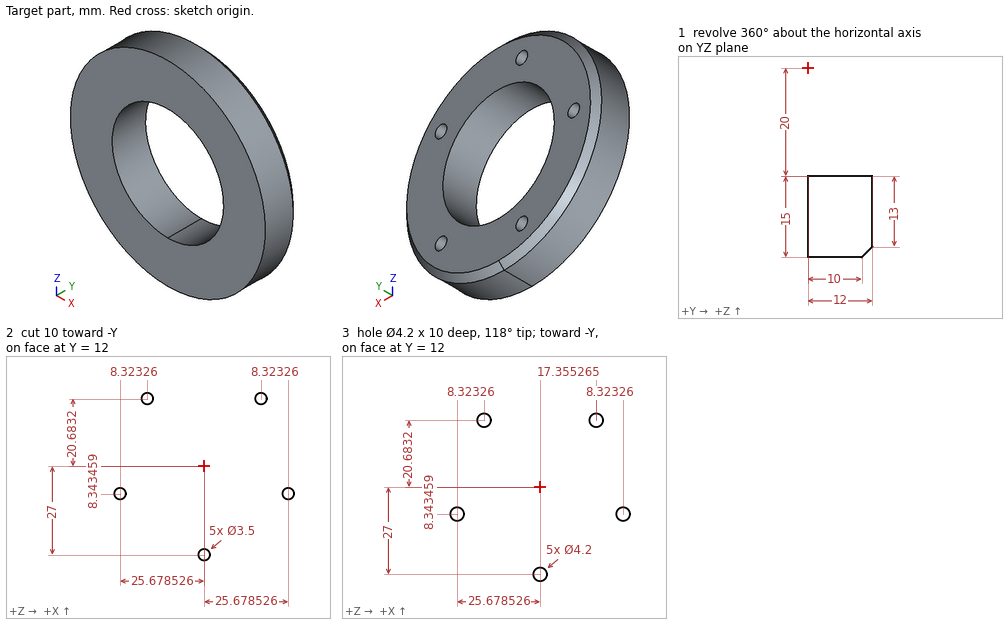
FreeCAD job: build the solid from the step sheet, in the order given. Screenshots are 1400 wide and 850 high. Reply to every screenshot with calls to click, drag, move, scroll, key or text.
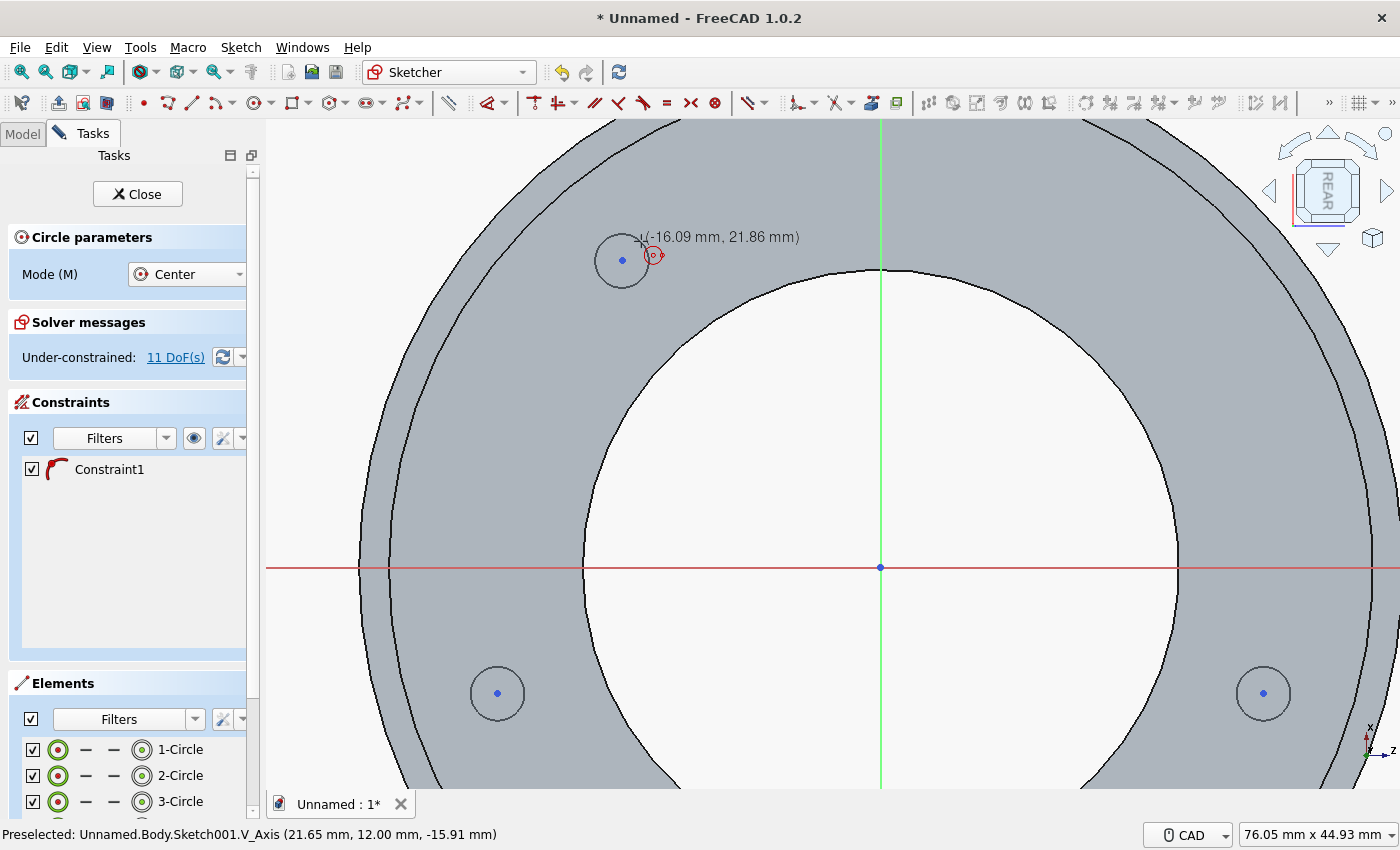
click(1140, 260)
click(1158, 241)
key(Escape)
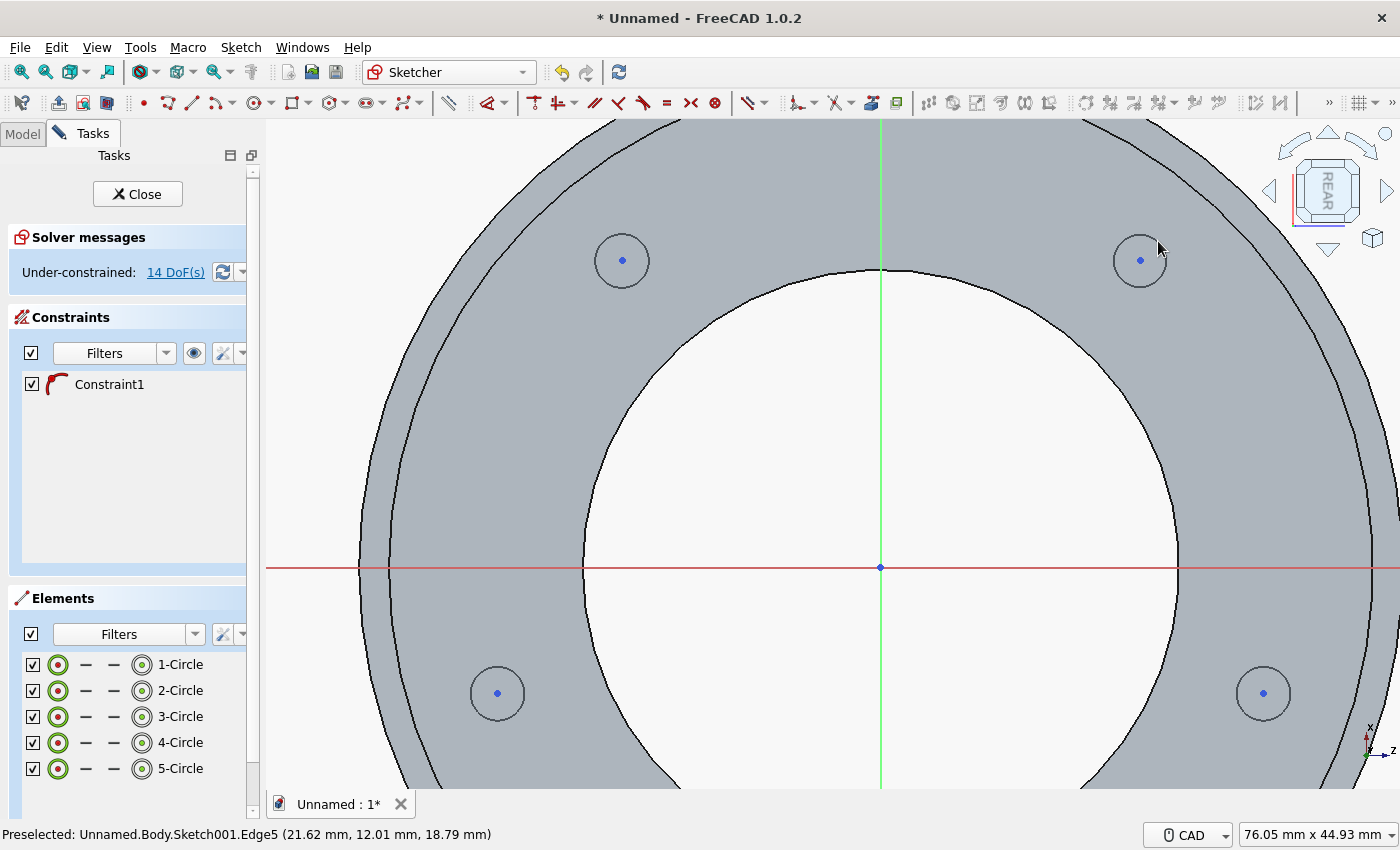
scroll(623, 258, down, 3)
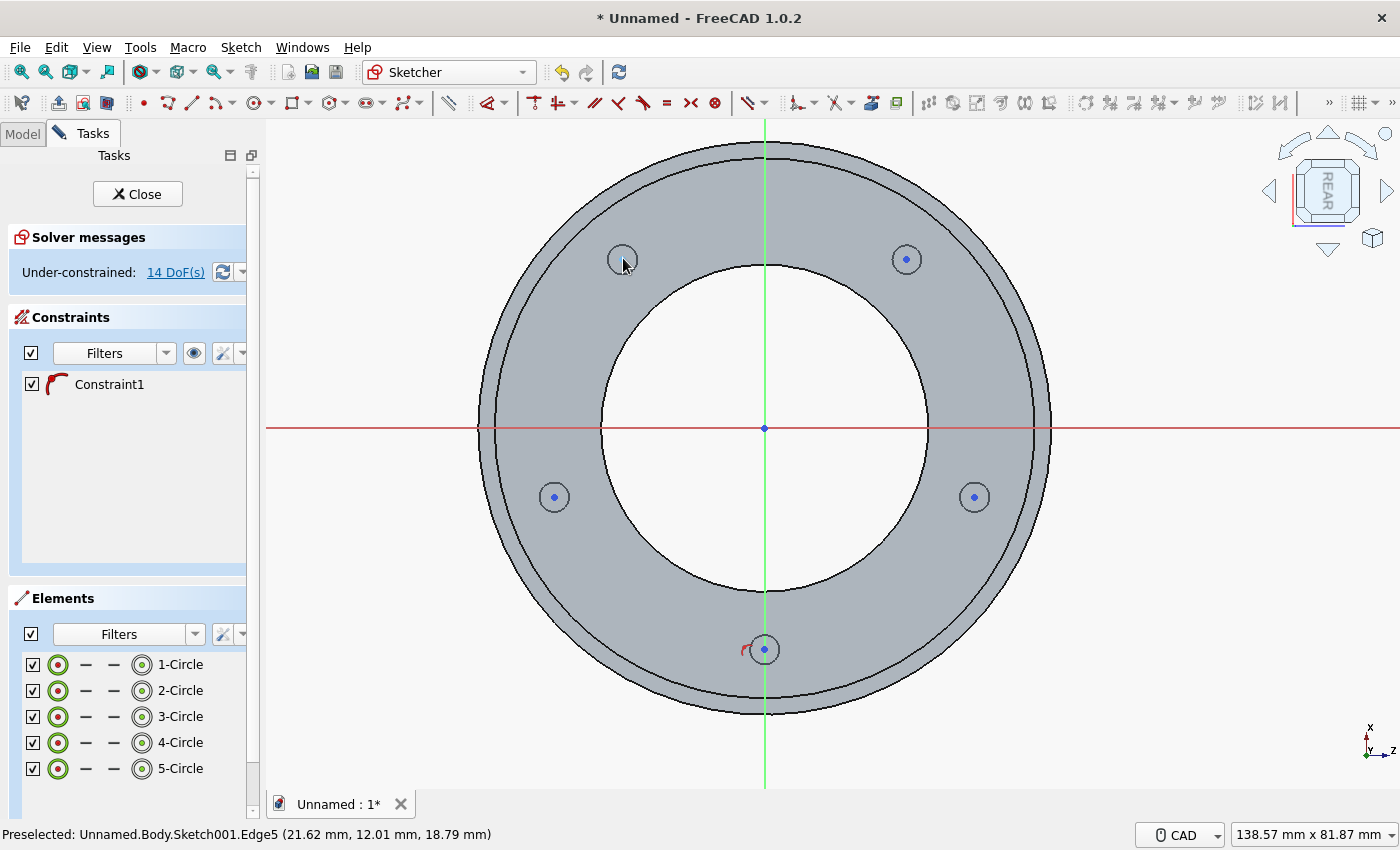
scroll(775, 639, up, 2)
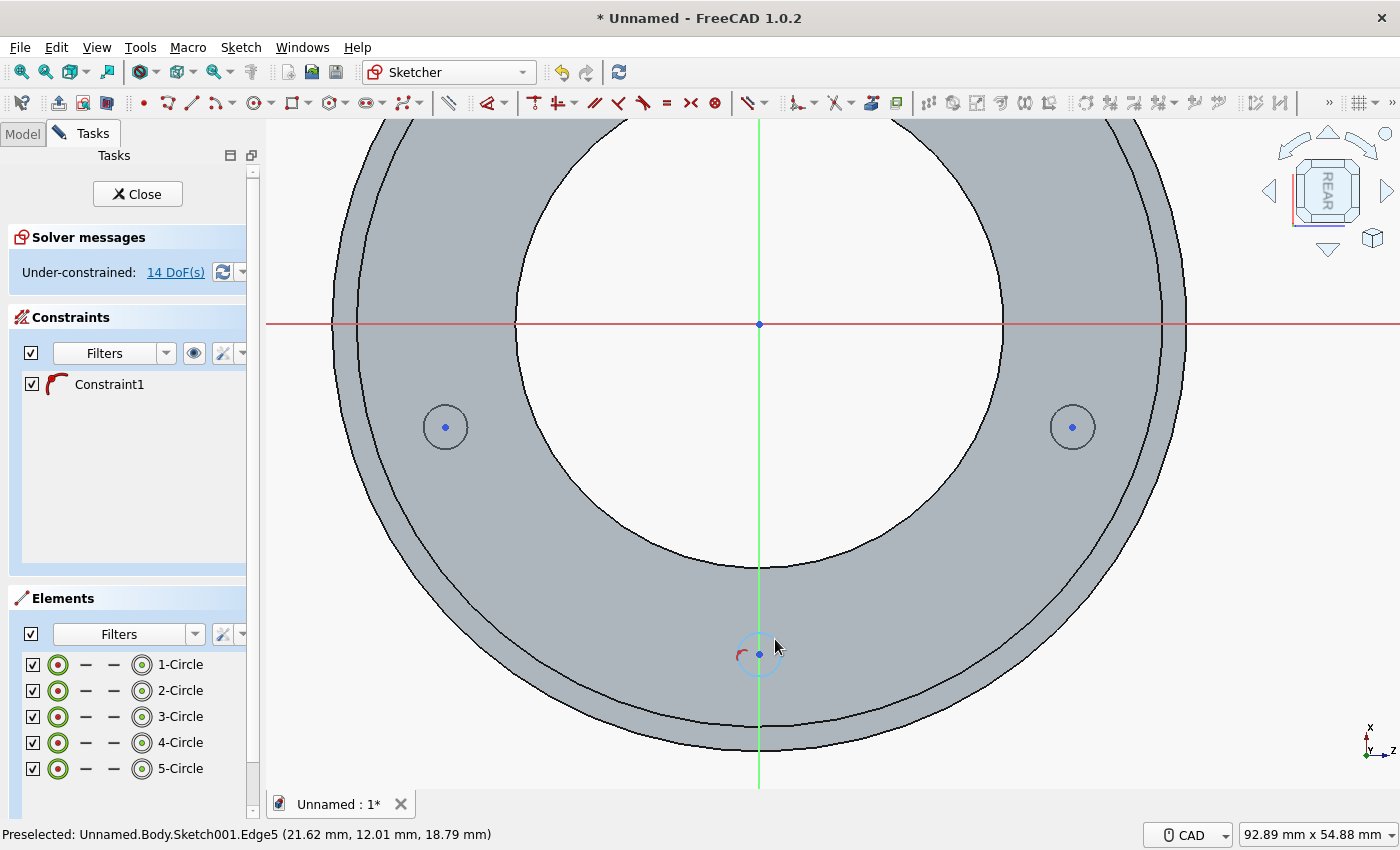
click(775, 639)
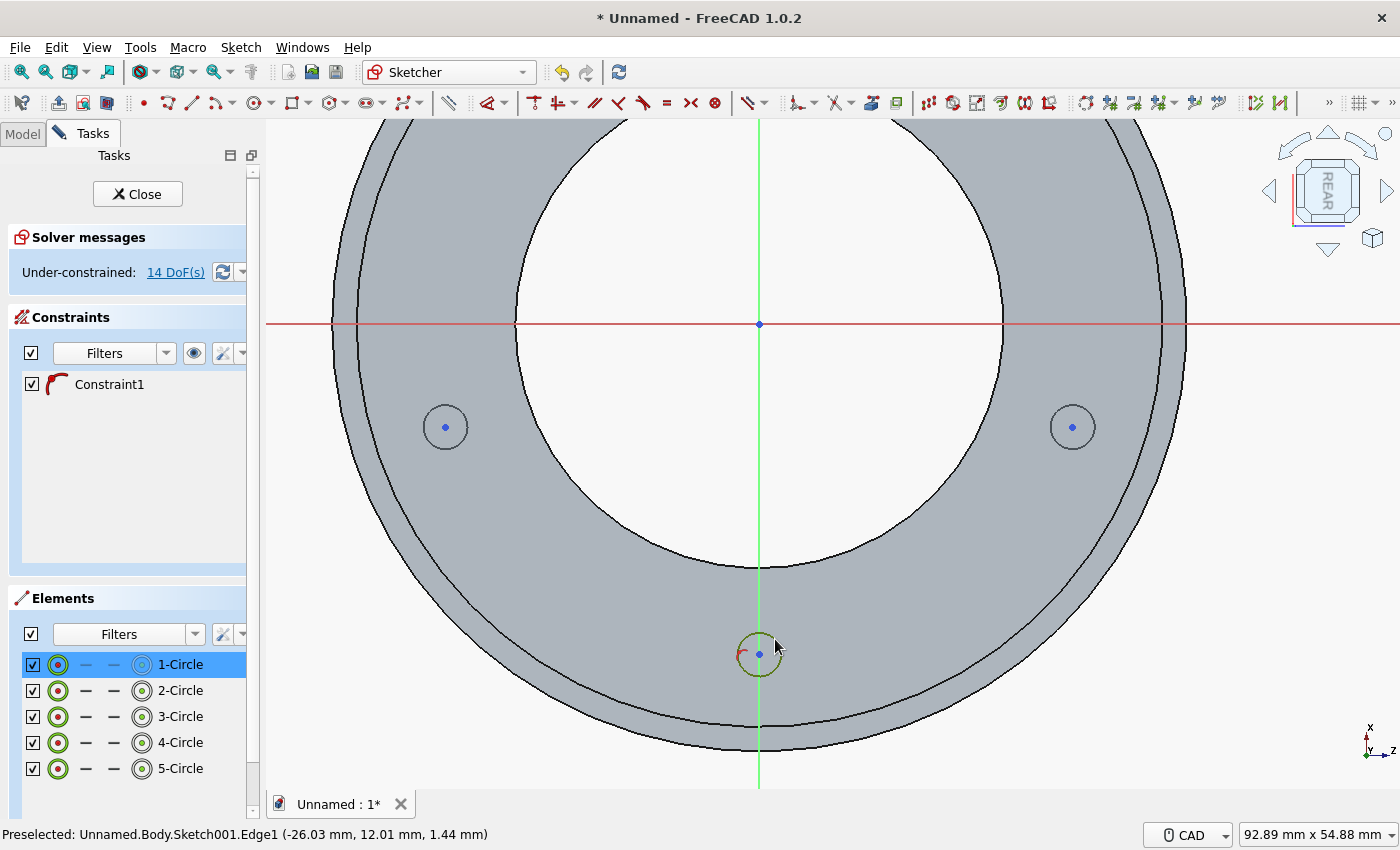
click(461, 412)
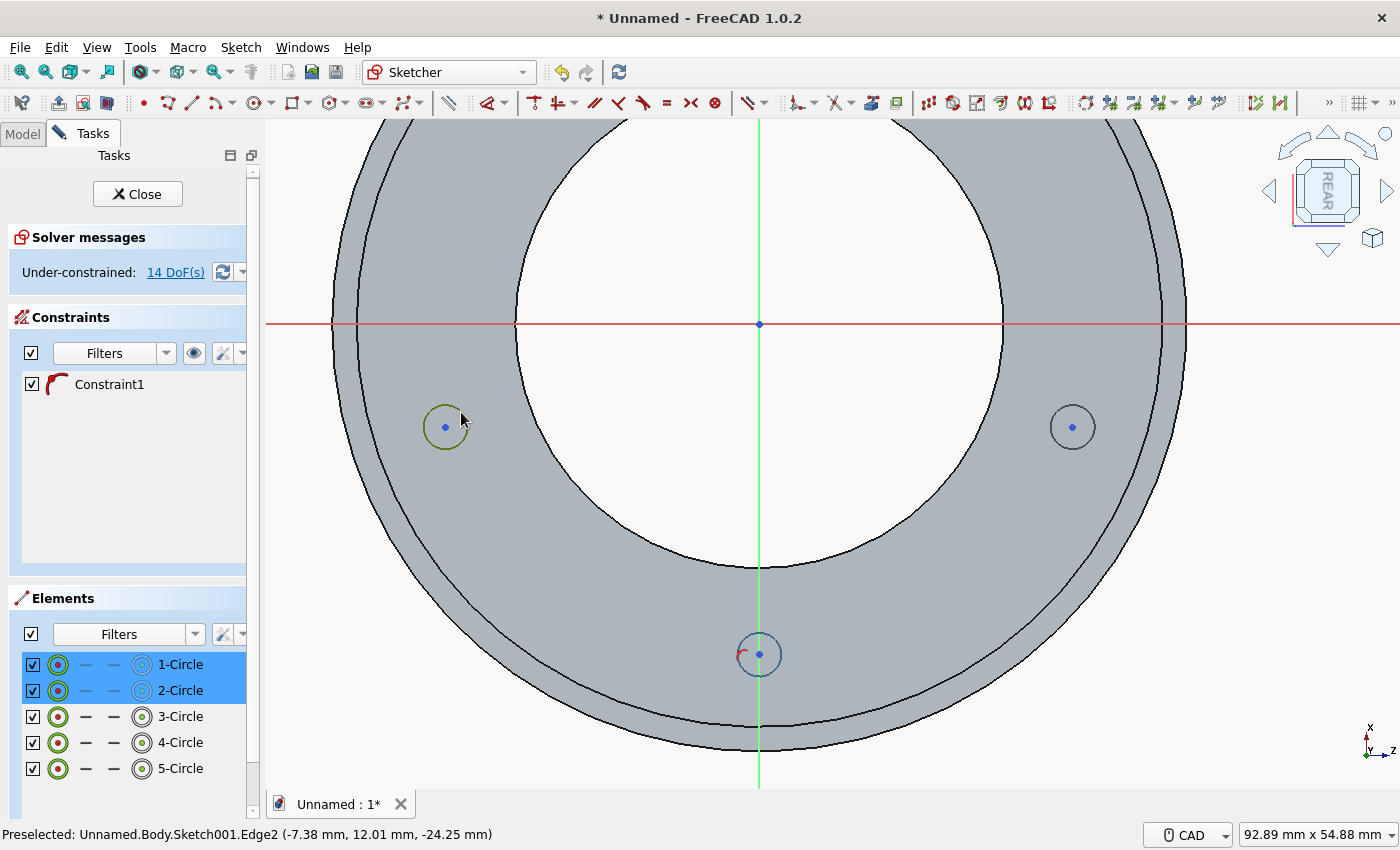
click(1088, 412)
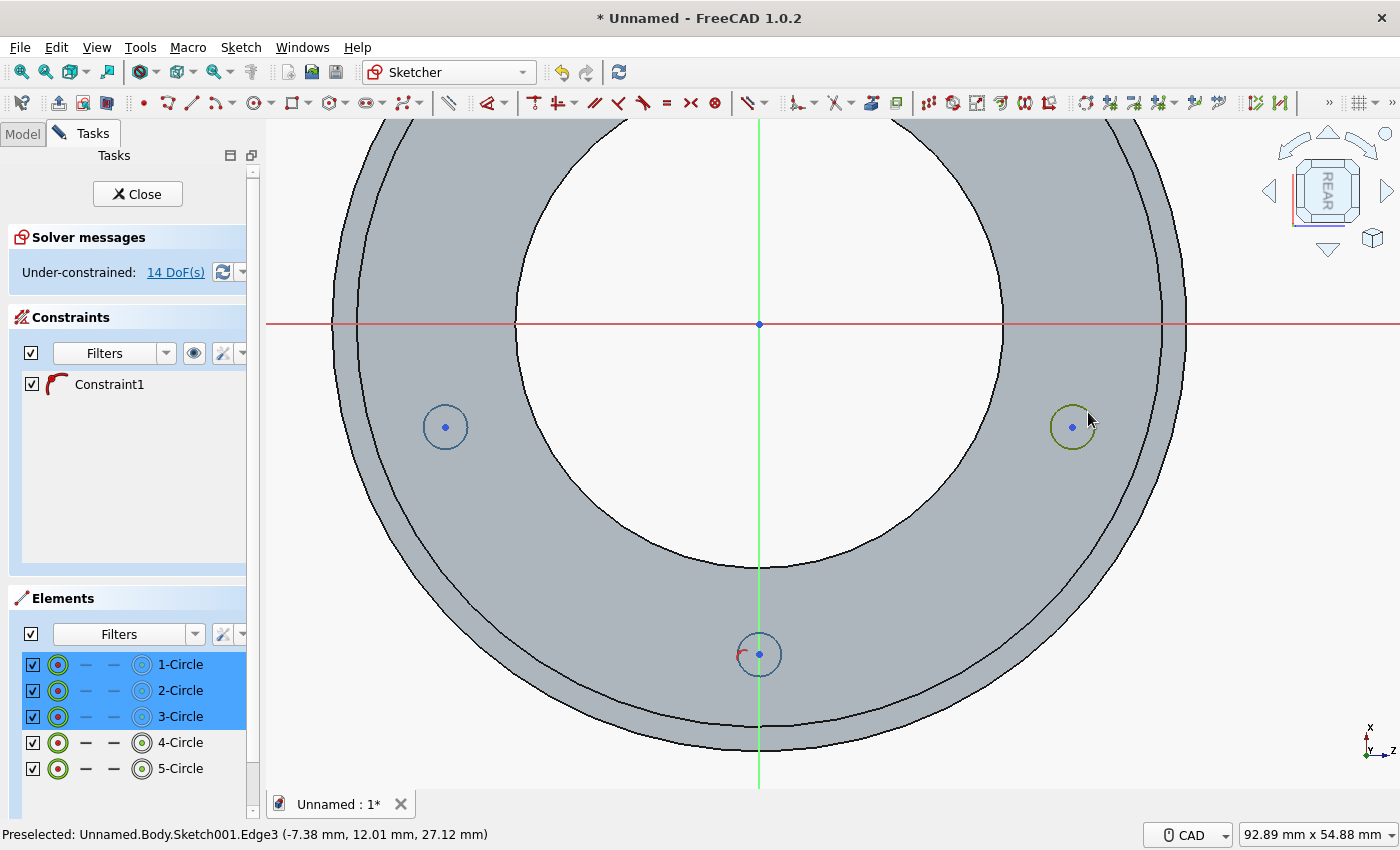
scroll(775, 640, down, 2)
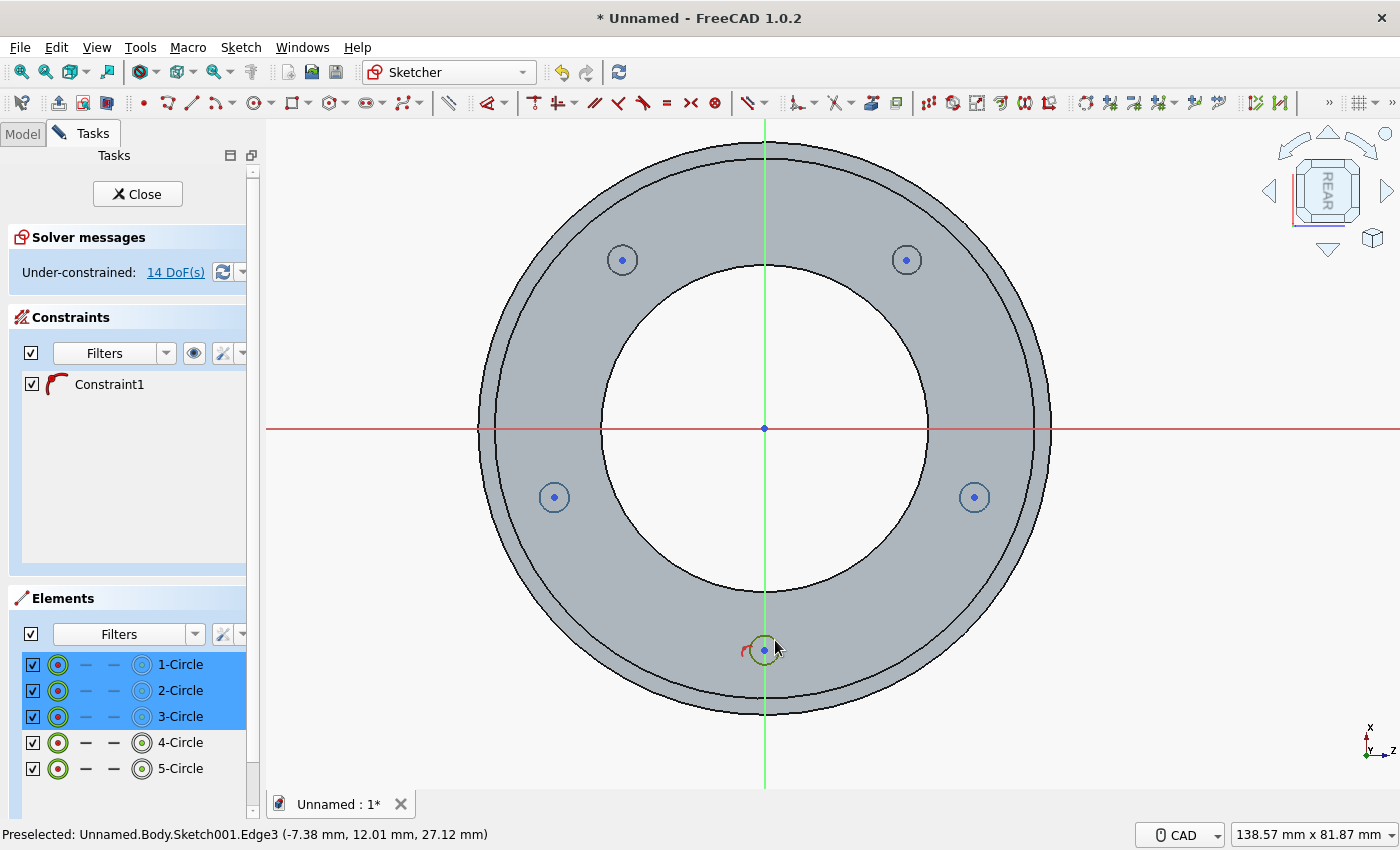
click(633, 250)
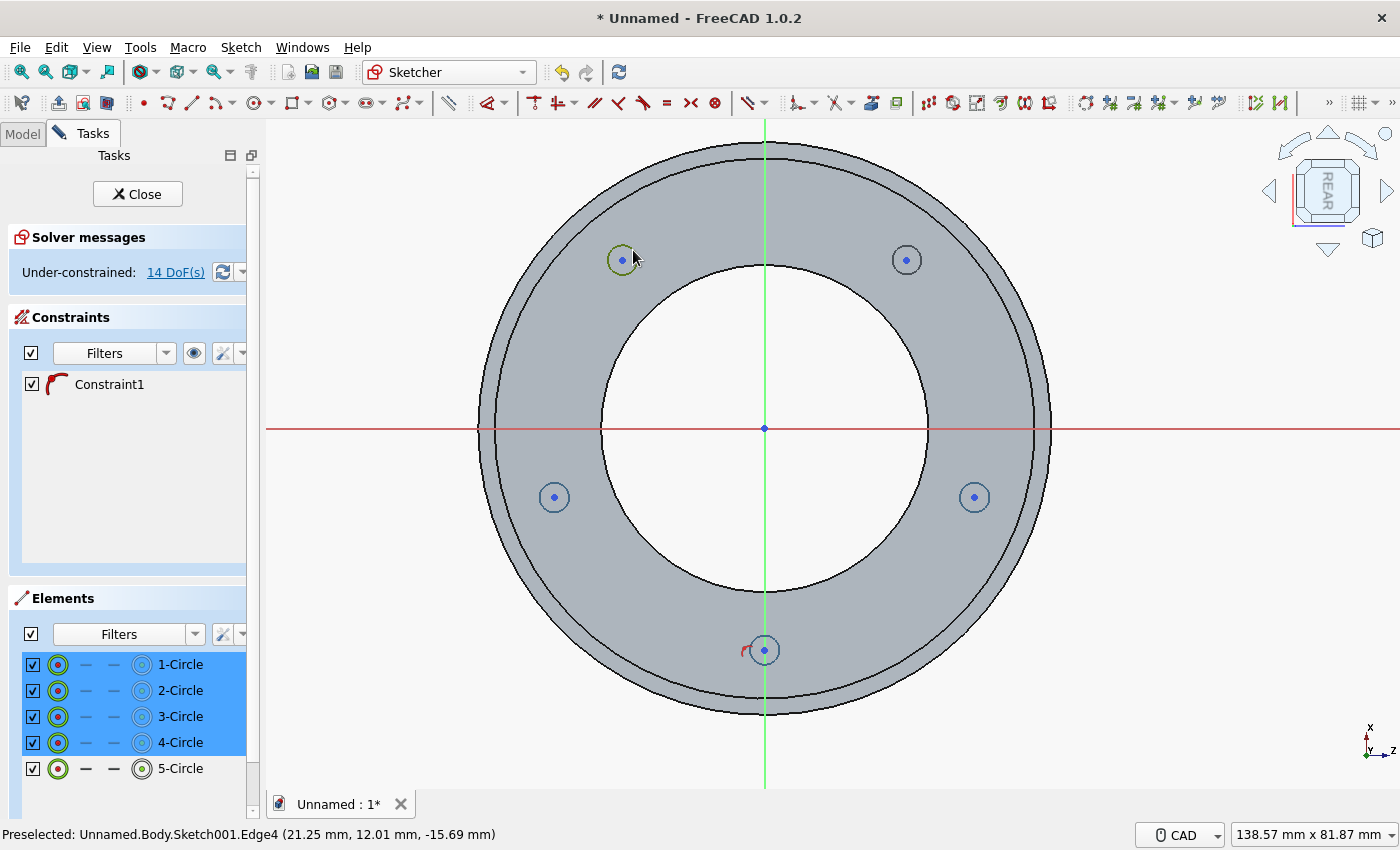
click(917, 250)